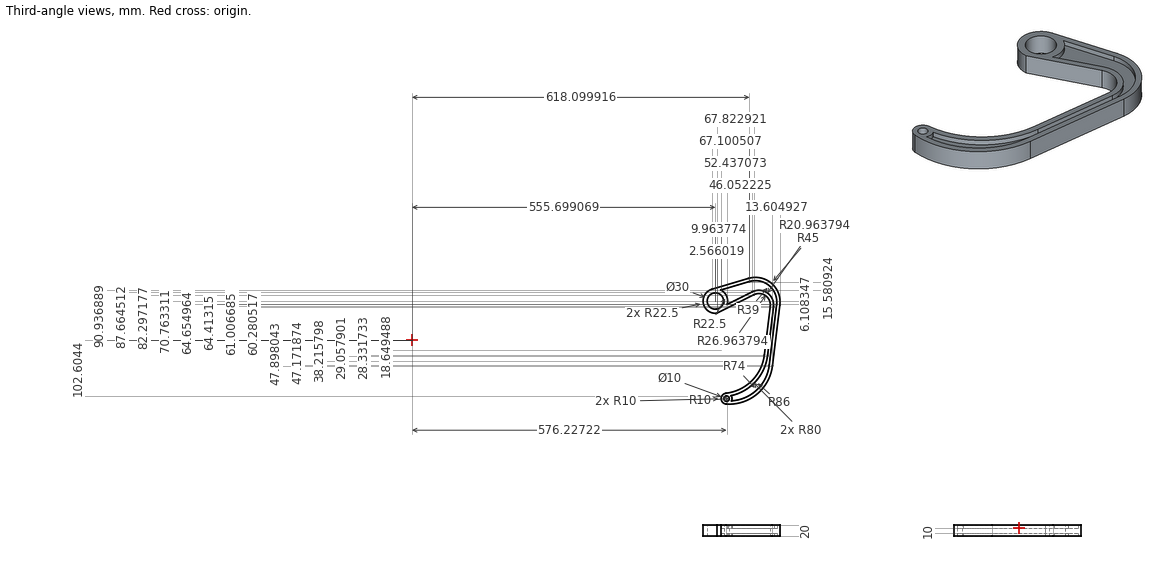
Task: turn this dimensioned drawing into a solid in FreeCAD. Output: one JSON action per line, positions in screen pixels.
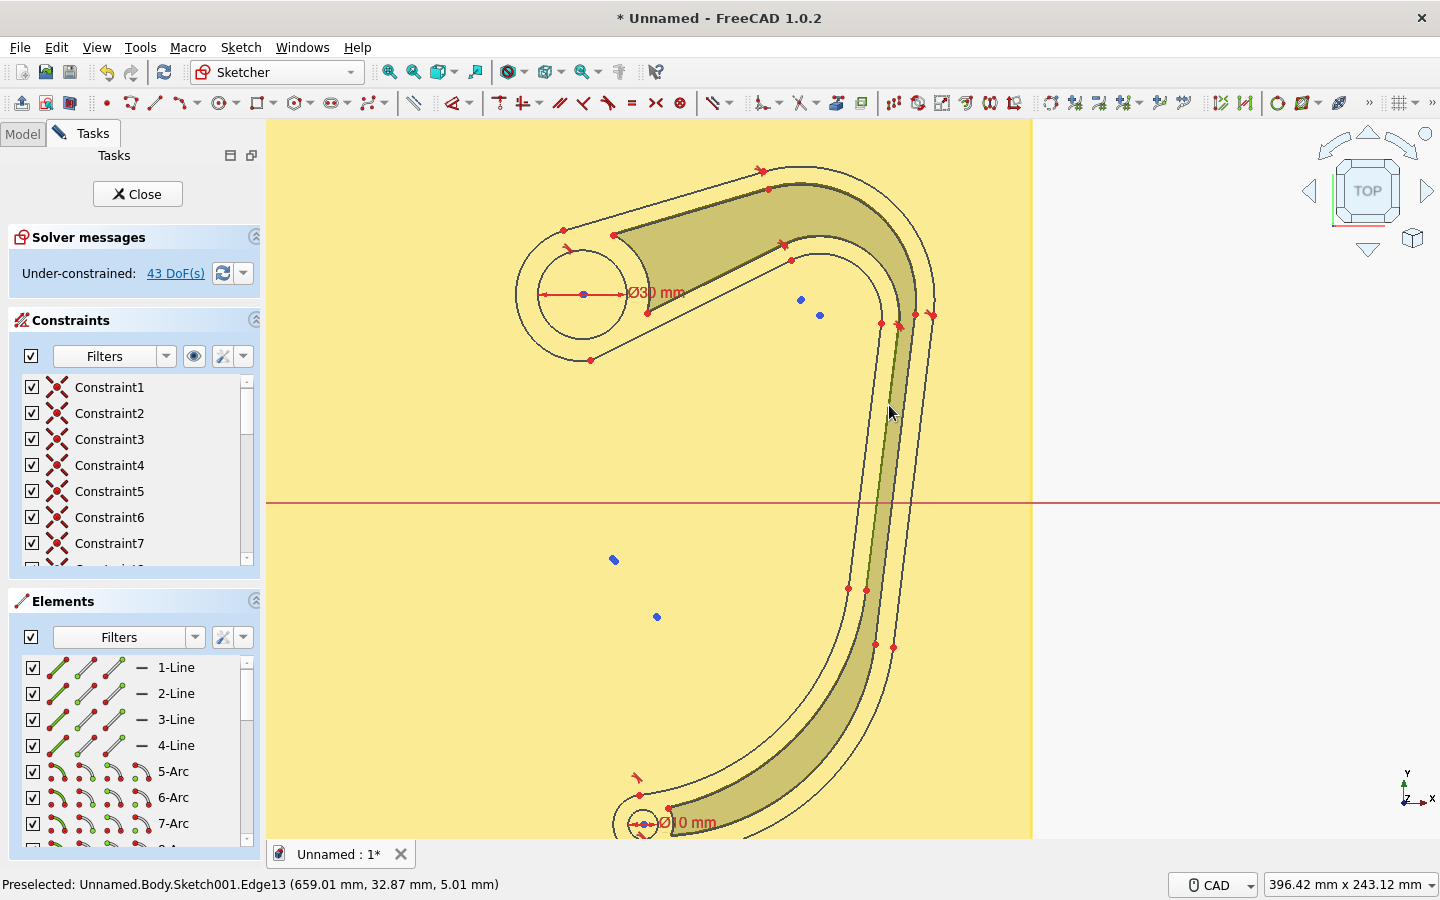
{"action": "left_click", "coordinate": [889, 276]}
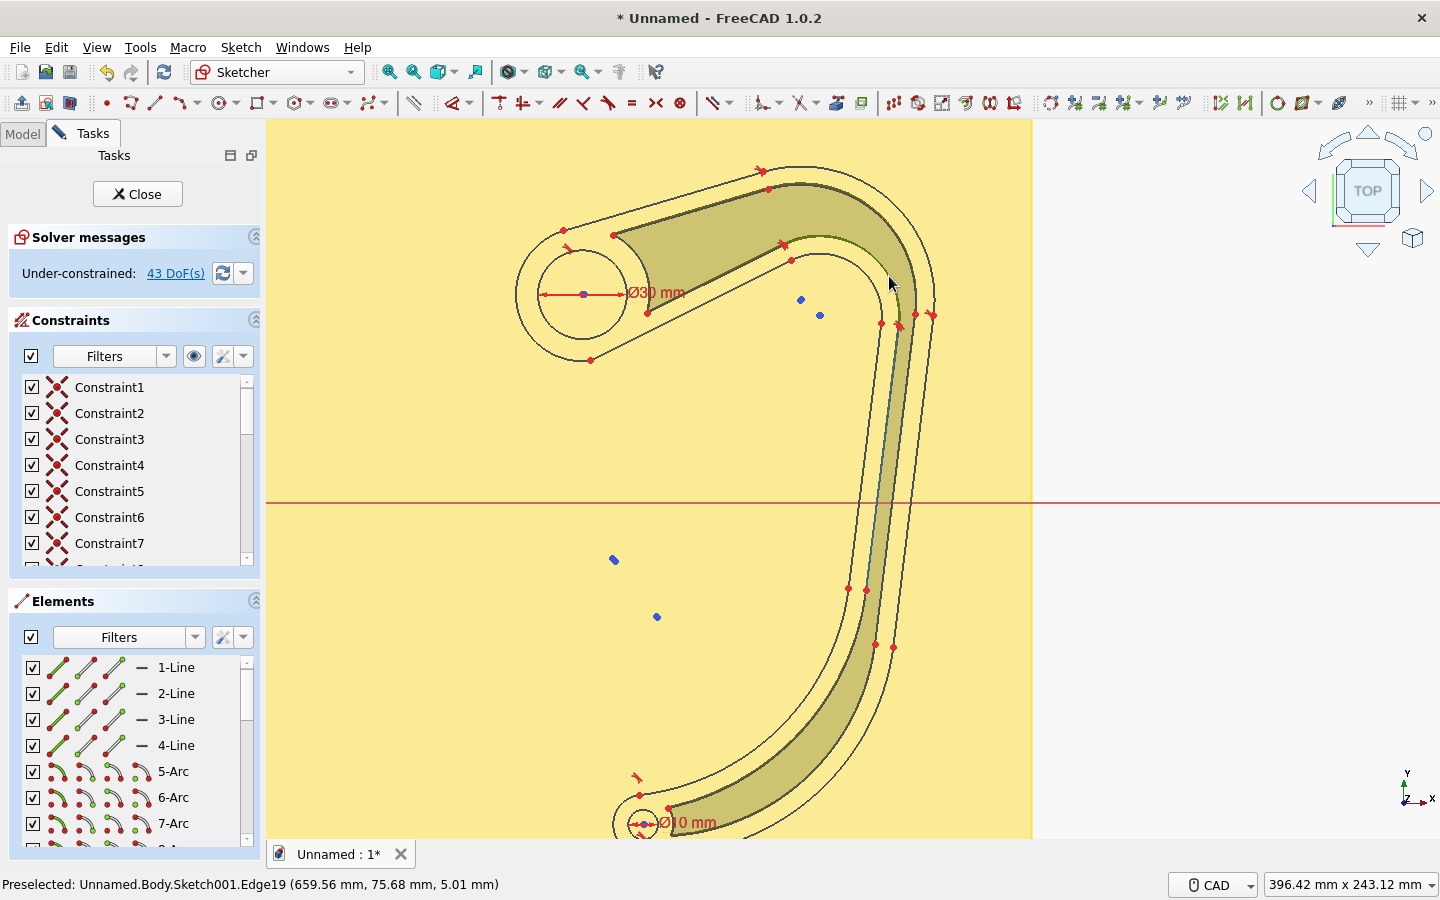
{"action": "left_click", "coordinate": [608, 104]}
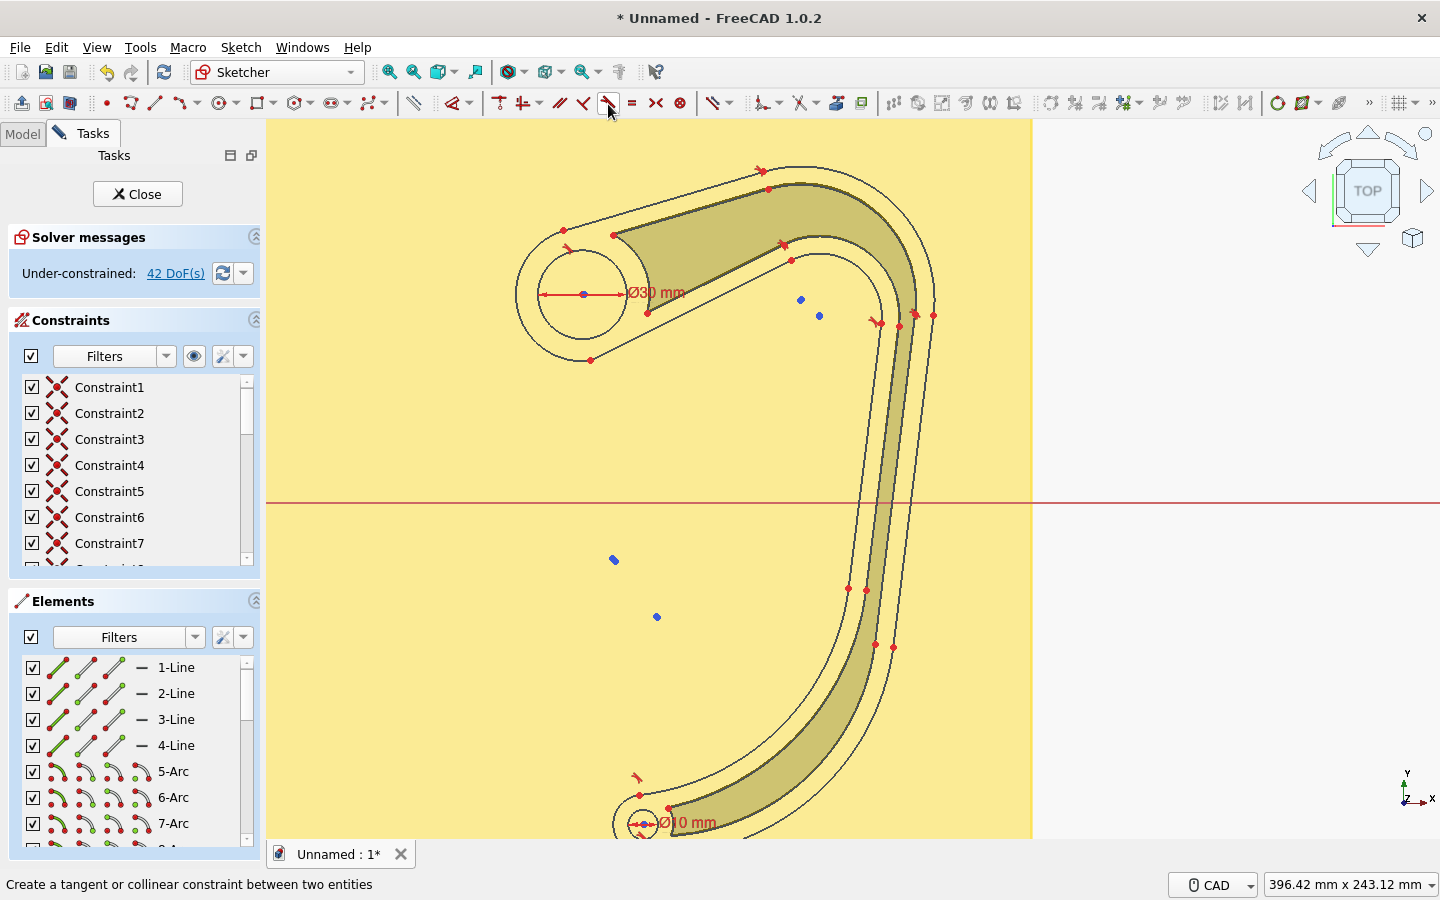
{"action": "left_click", "coordinate": [743, 265]}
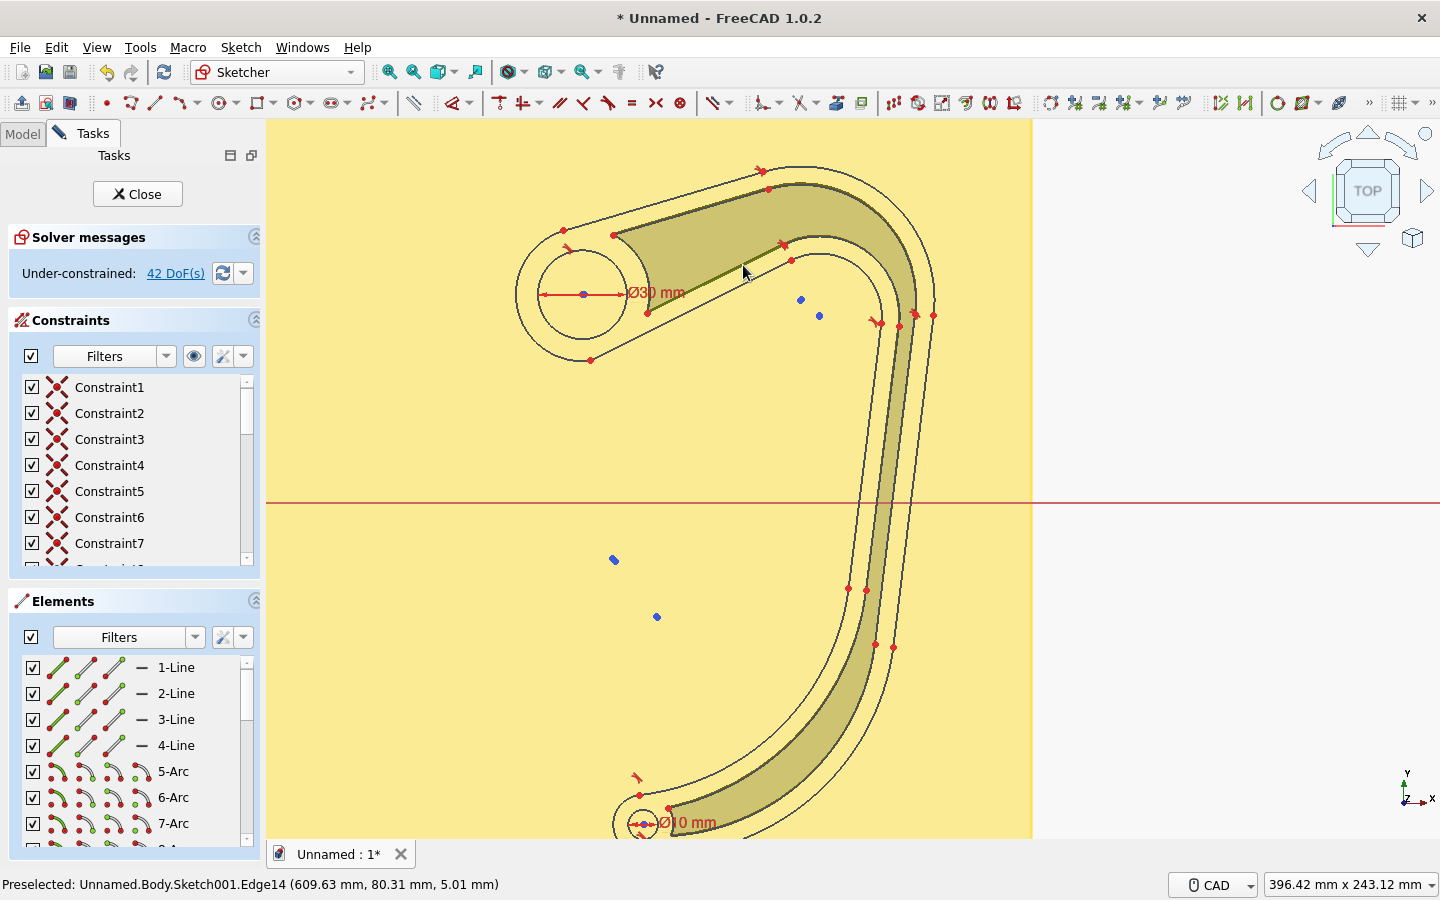
{"action": "left_click", "coordinate": [889, 276]}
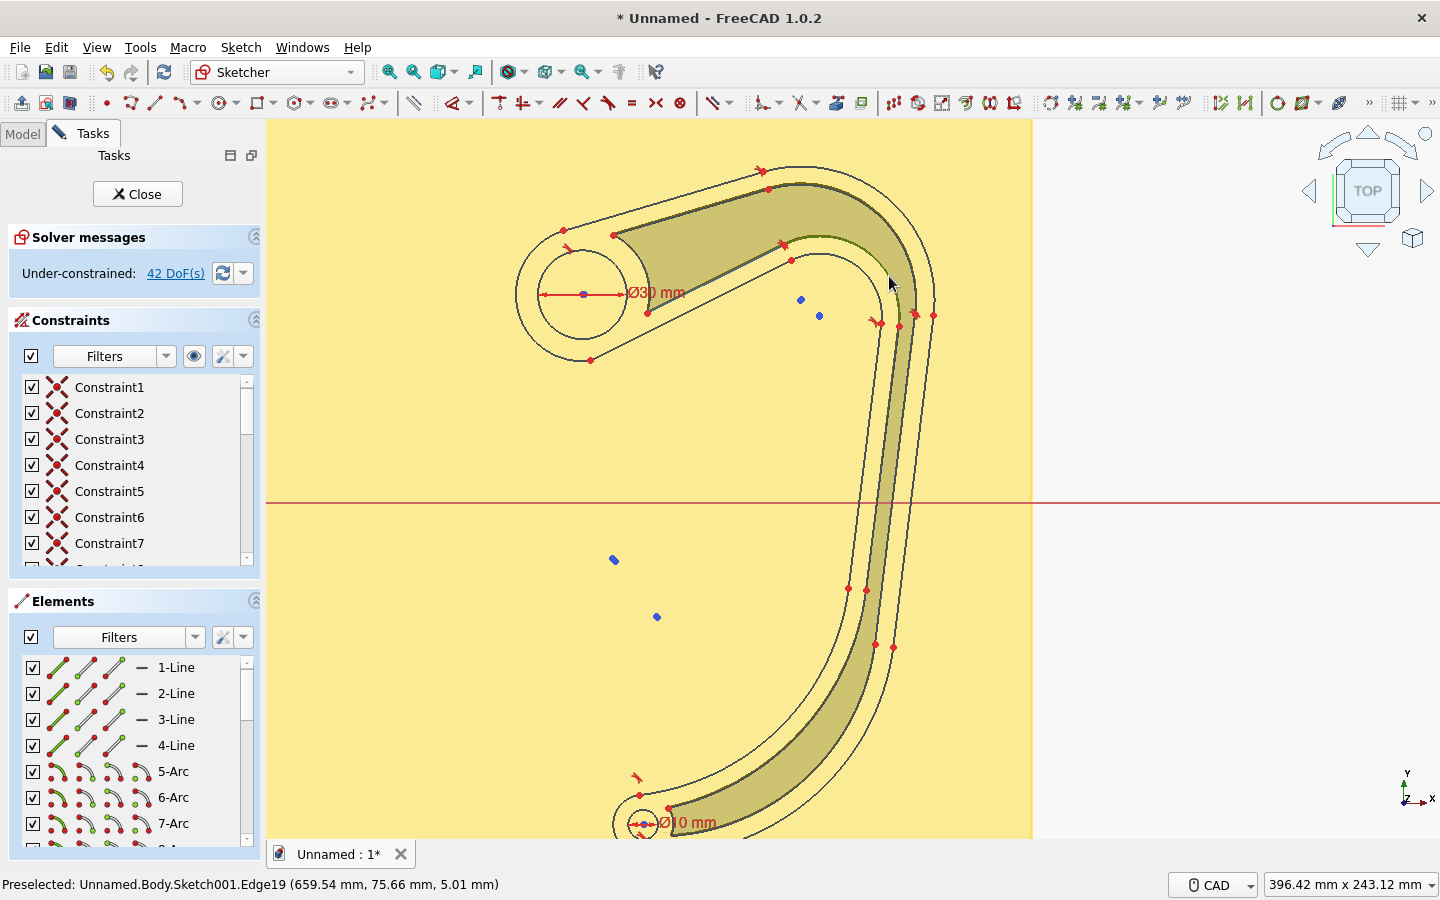
{"action": "left_click", "coordinate": [608, 104]}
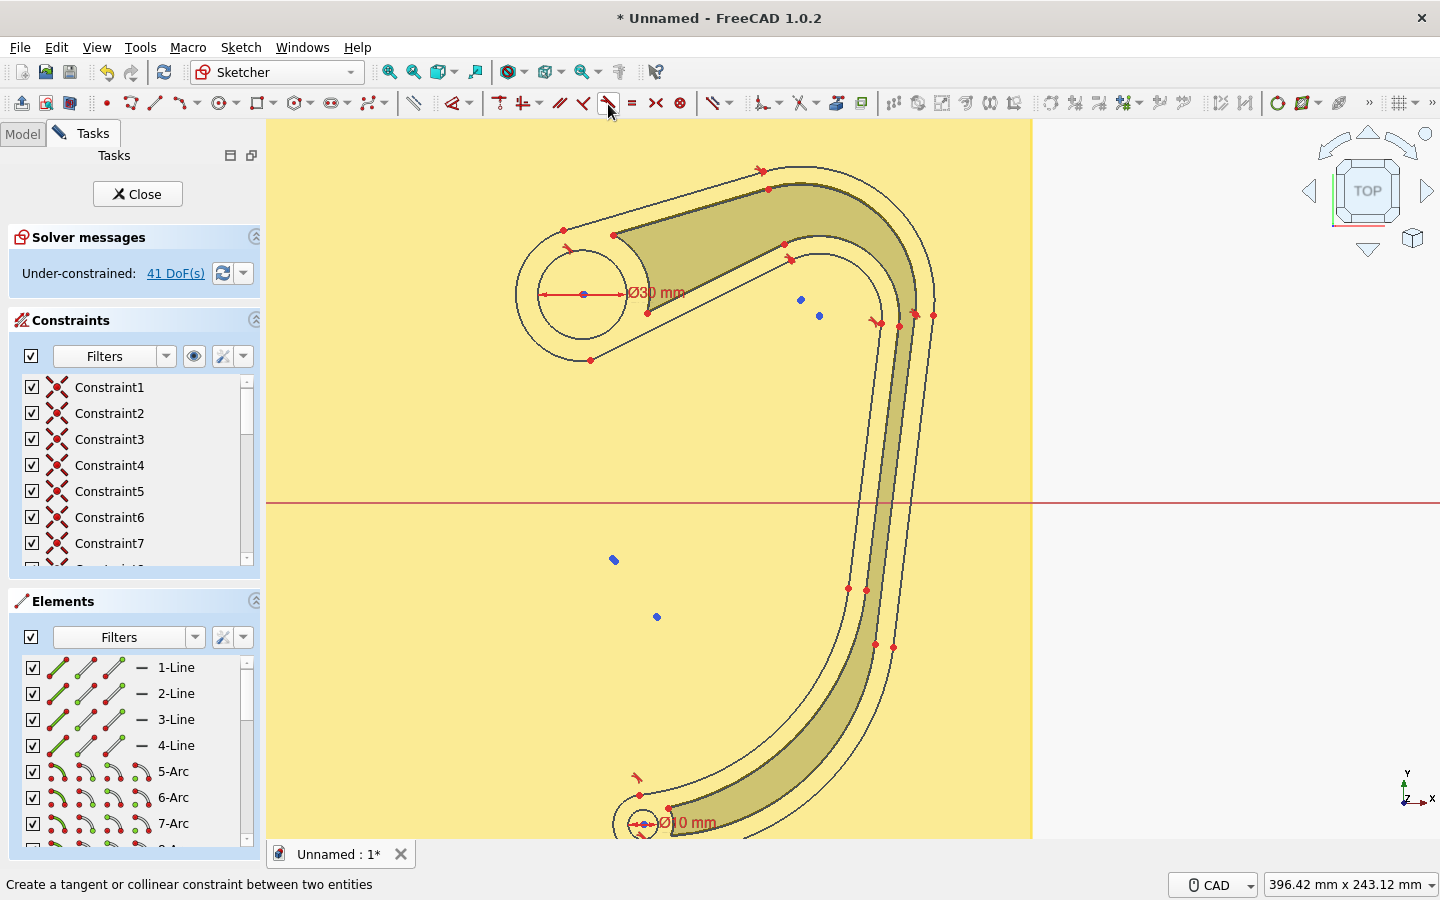
{"action": "left_click", "coordinate": [920, 239]}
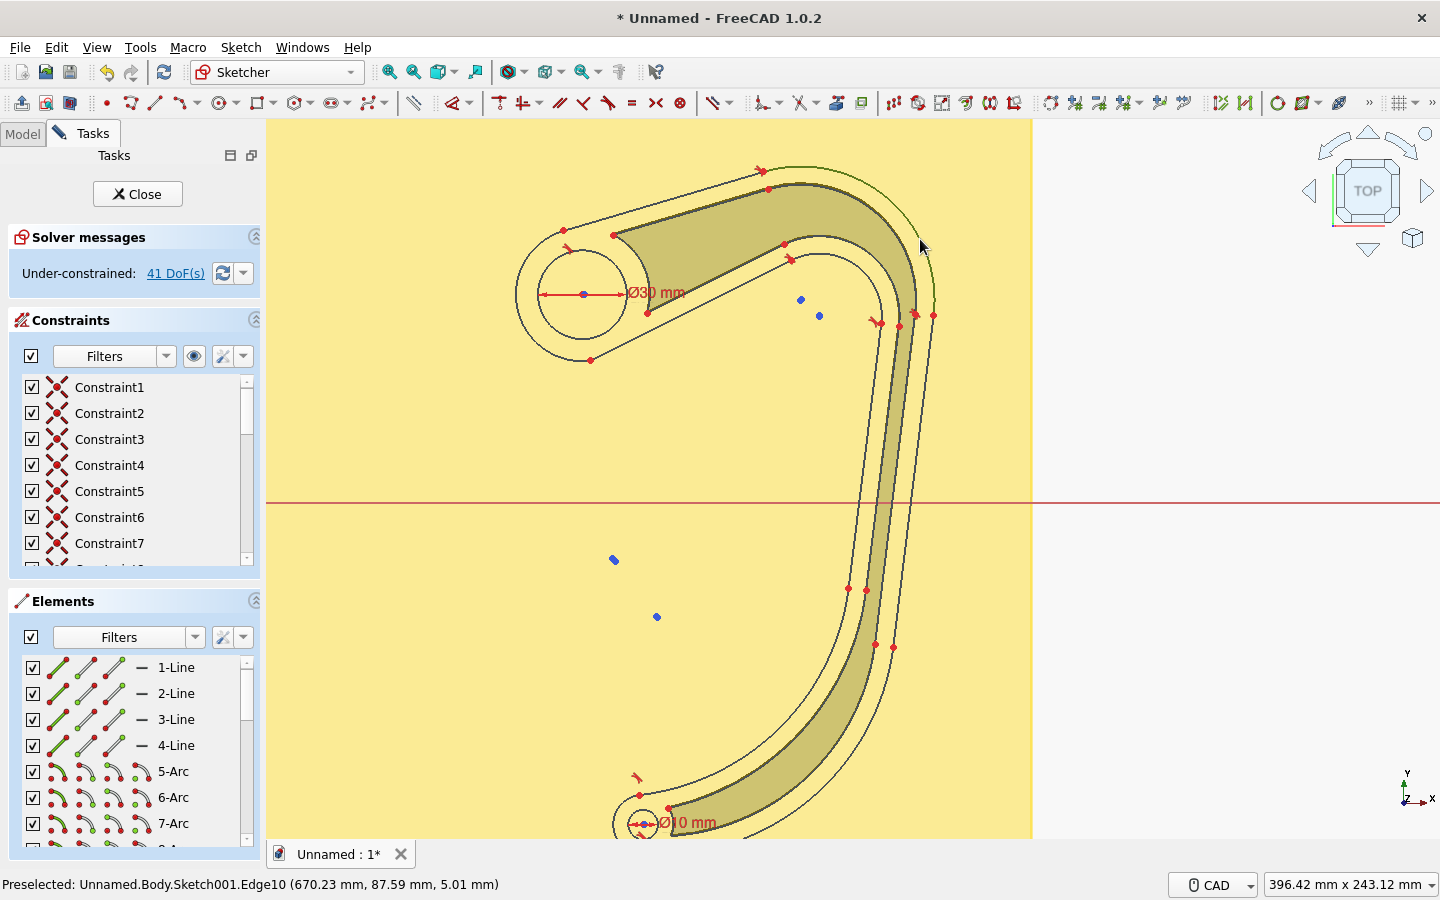
{"action": "left_click", "coordinate": [903, 248]}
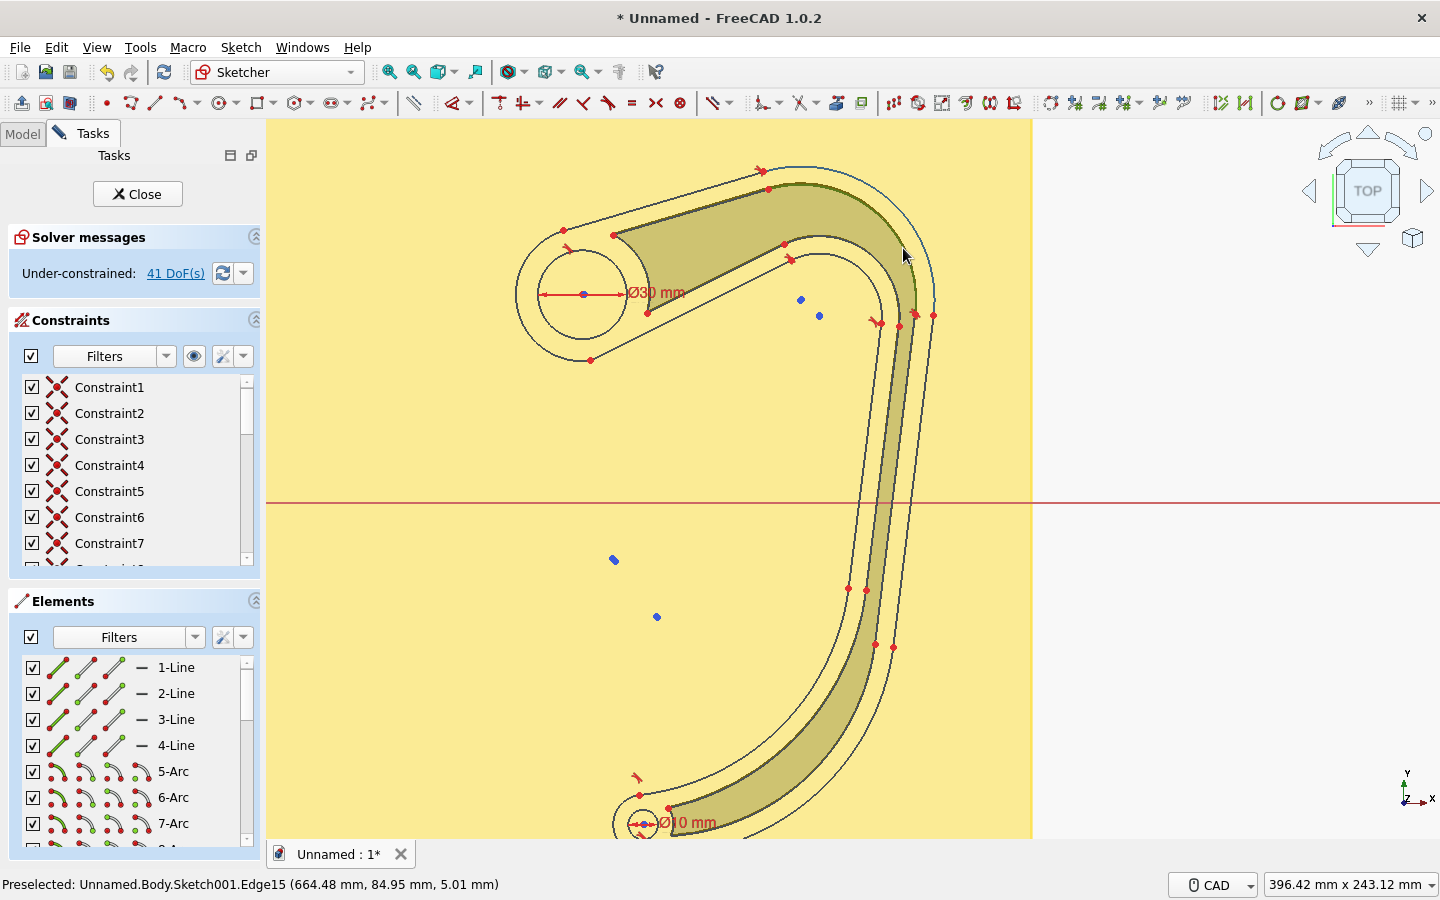
{"action": "key", "text": "c"}